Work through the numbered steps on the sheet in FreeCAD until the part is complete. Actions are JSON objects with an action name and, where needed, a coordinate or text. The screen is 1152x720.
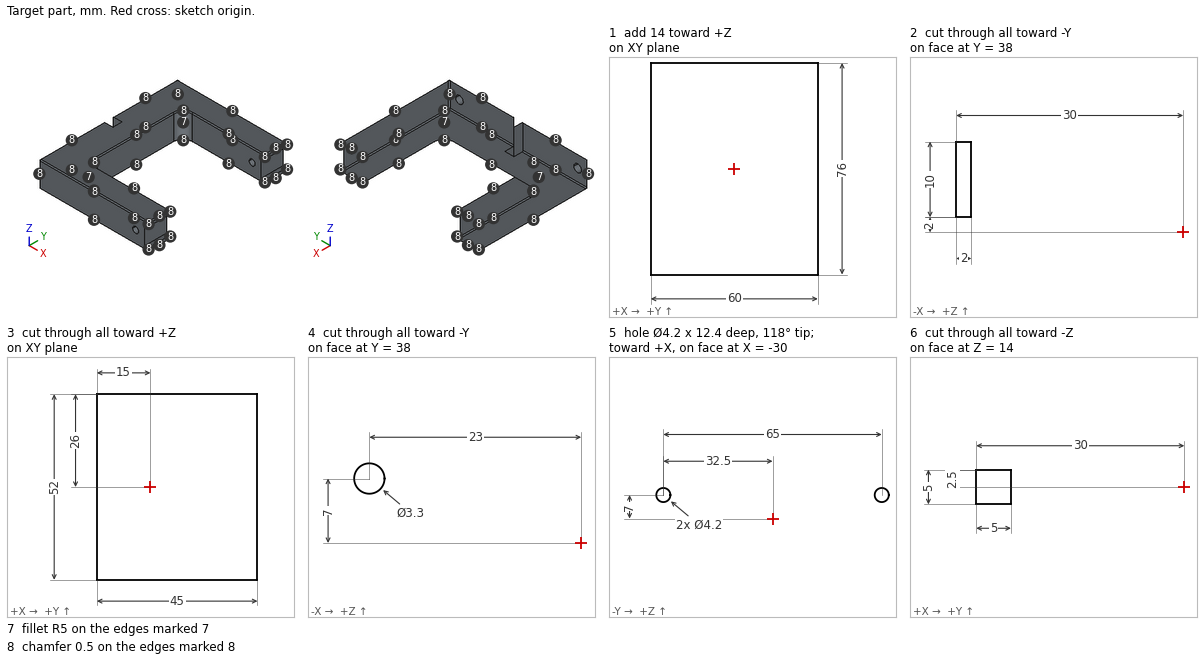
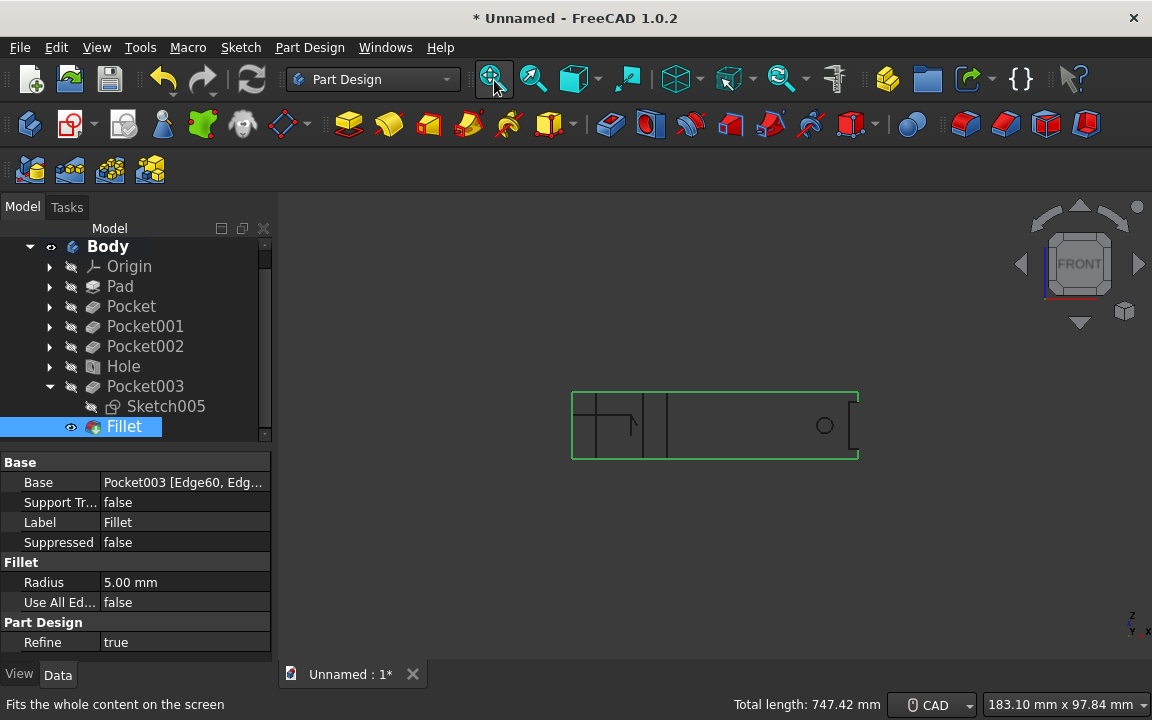
{"action": "key", "text": "3"}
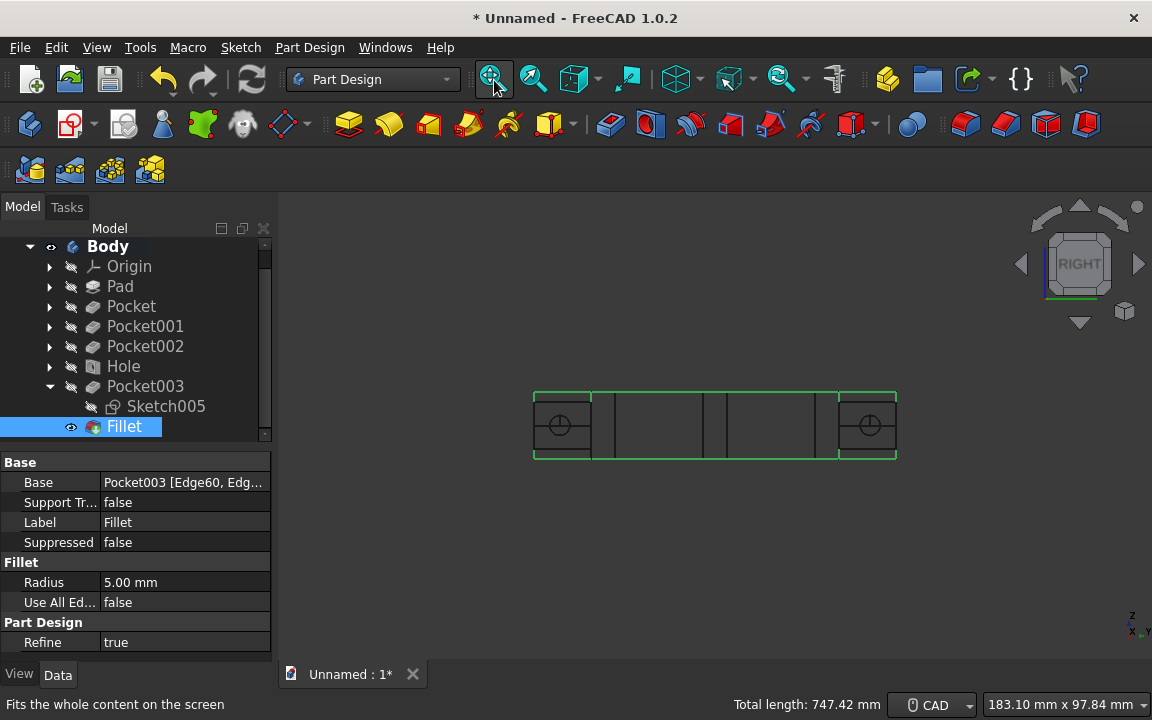
{"action": "key", "text": "v f"}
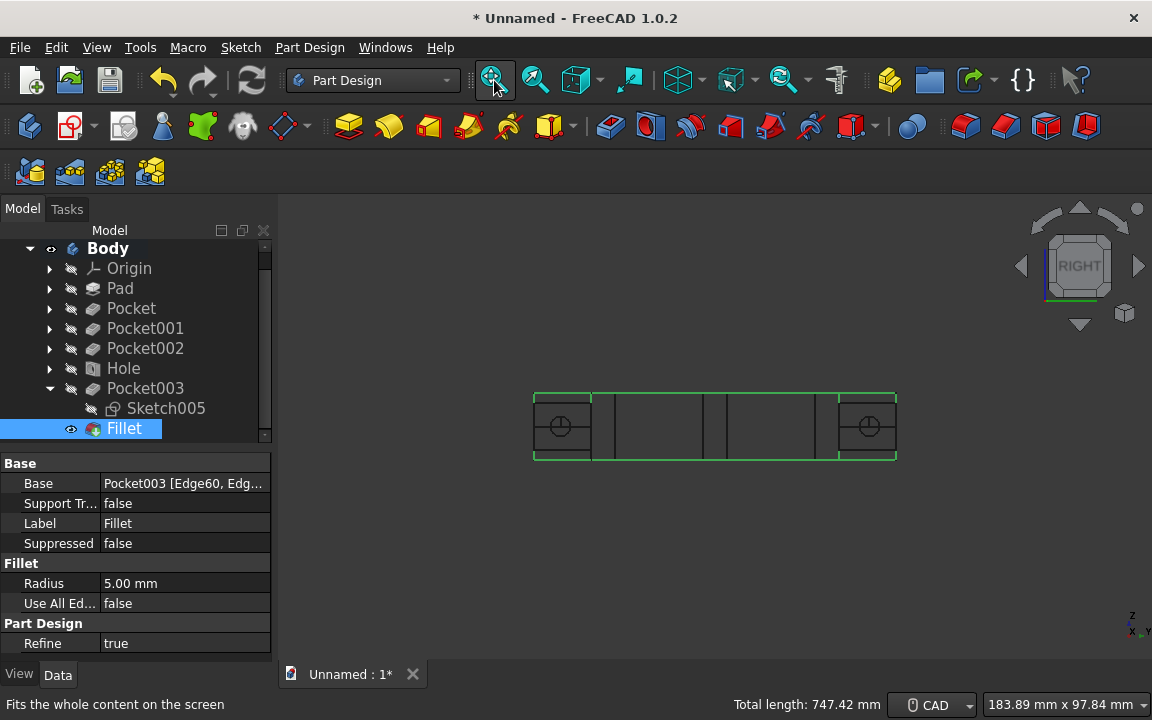
{"action": "left_click", "coordinate": [591, 452], "text": "ctrl"}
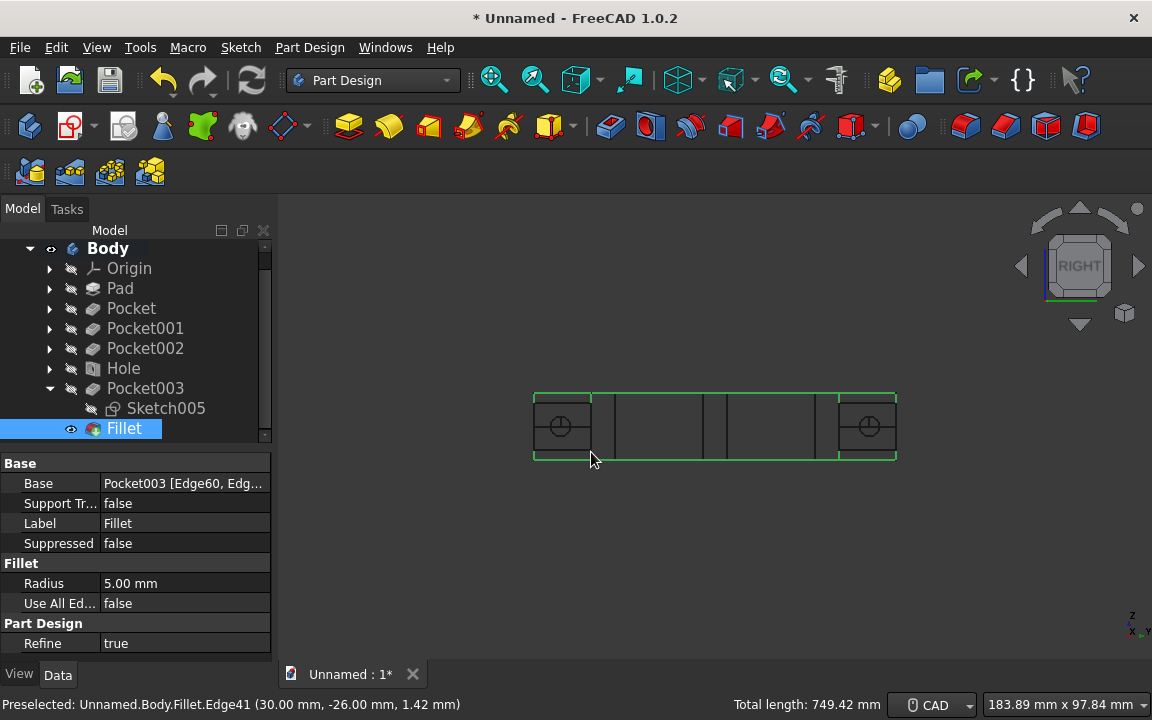
{"action": "key", "text": "v 1"}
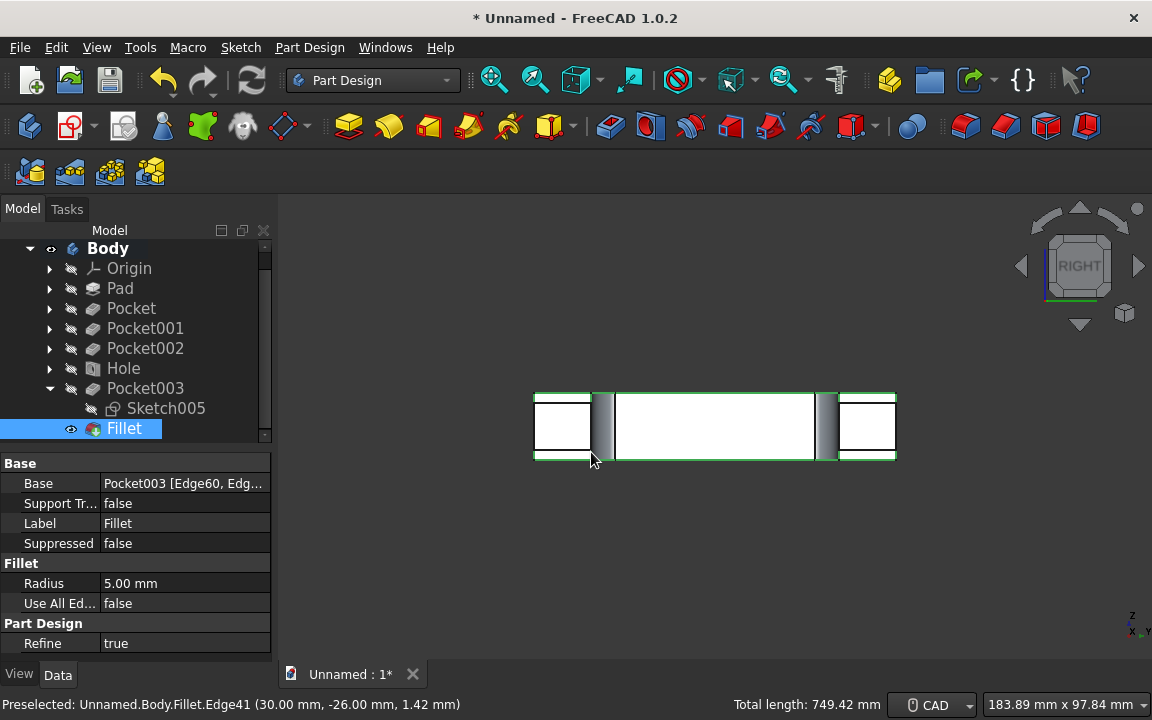
{"action": "left_click", "coordinate": [1006, 126]}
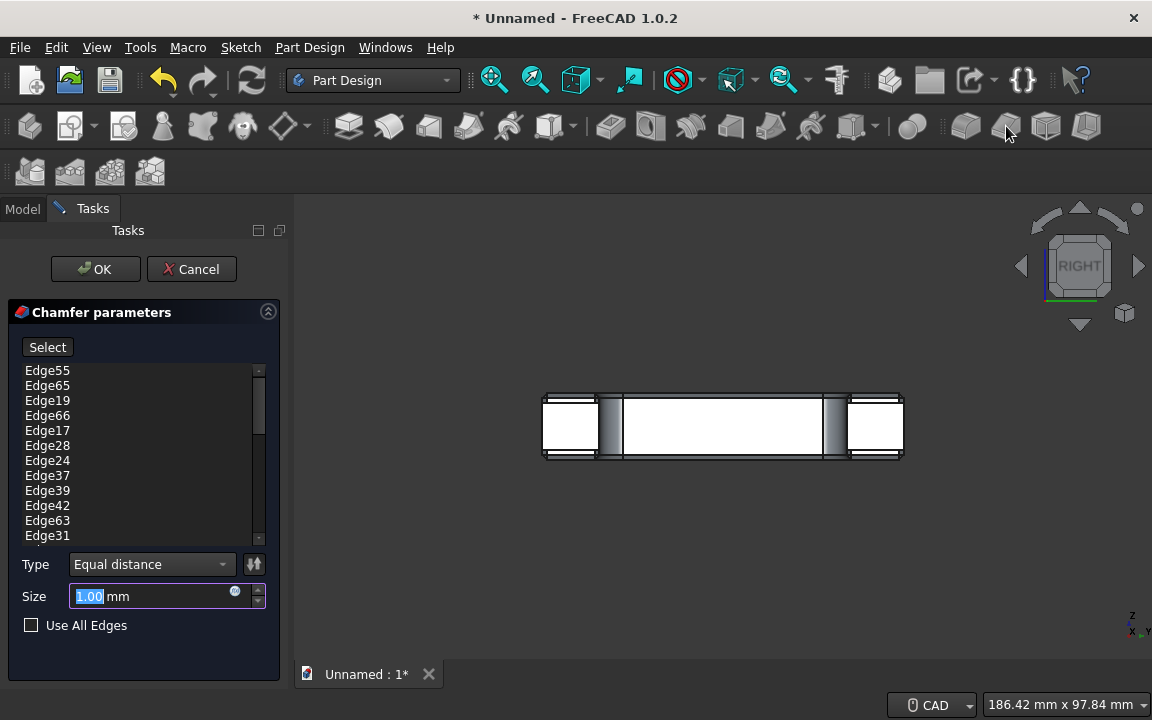
{"action": "type", "text": "0.5"}
{"action": "key", "text": "Tab"}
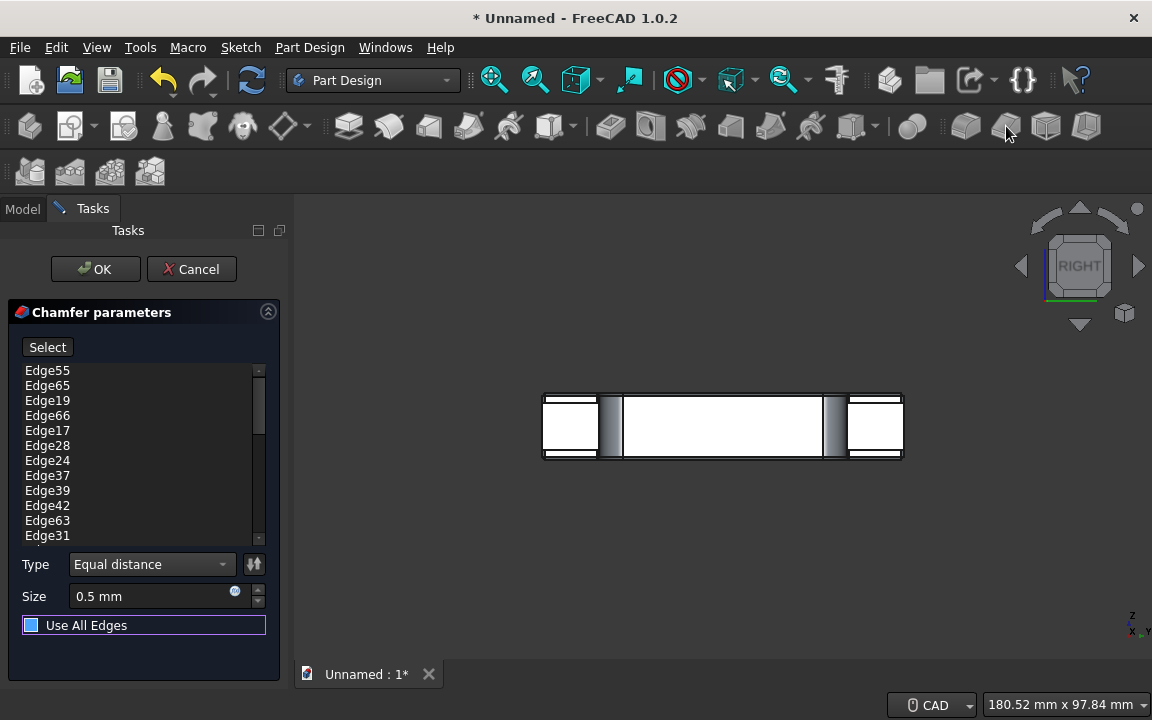
{"action": "left_click", "coordinate": [96, 269]}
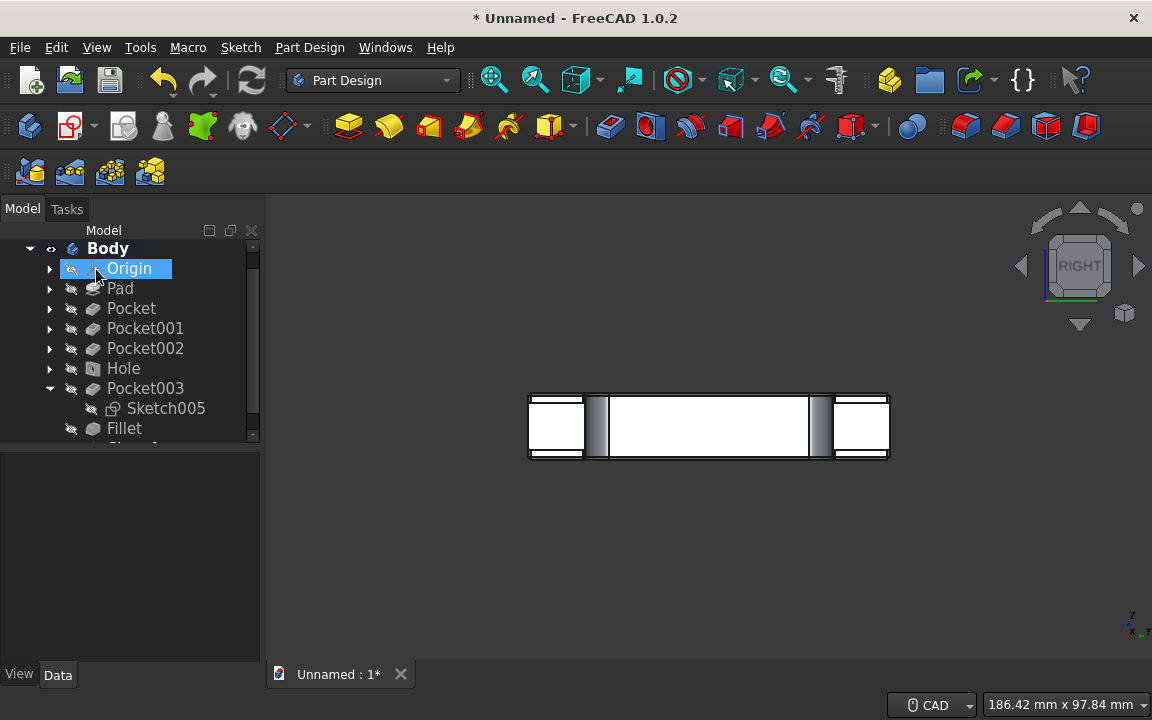
{"action": "key", "text": "0"}